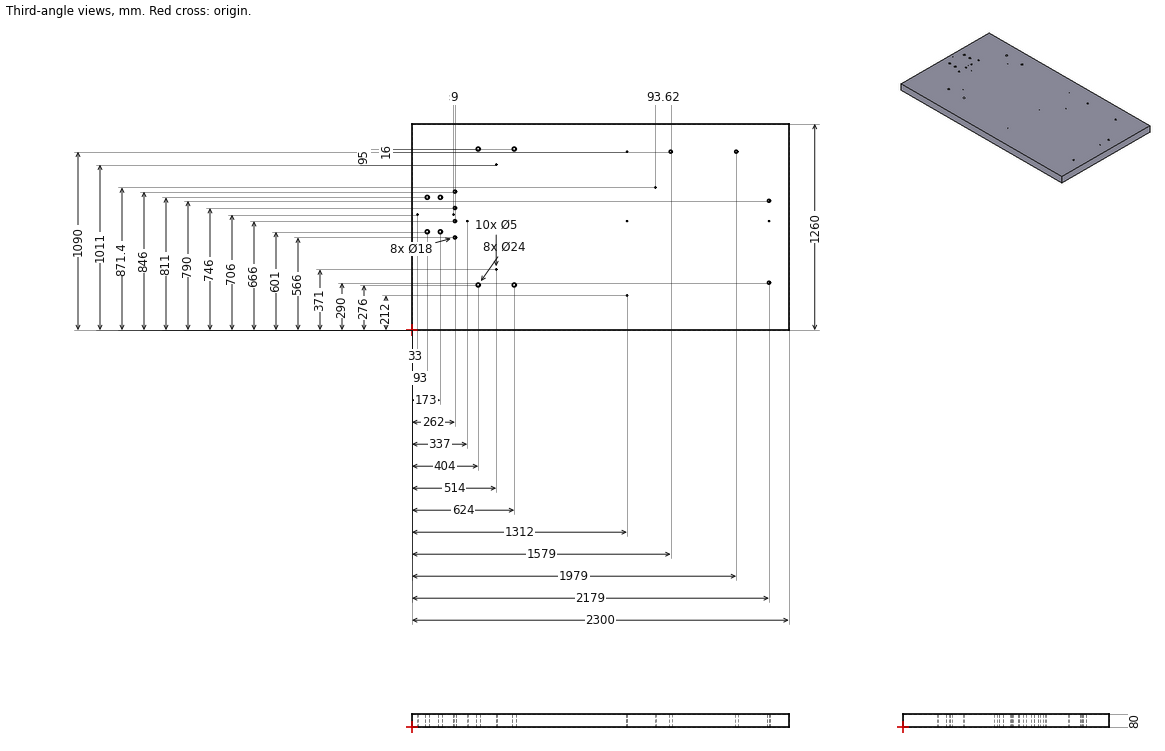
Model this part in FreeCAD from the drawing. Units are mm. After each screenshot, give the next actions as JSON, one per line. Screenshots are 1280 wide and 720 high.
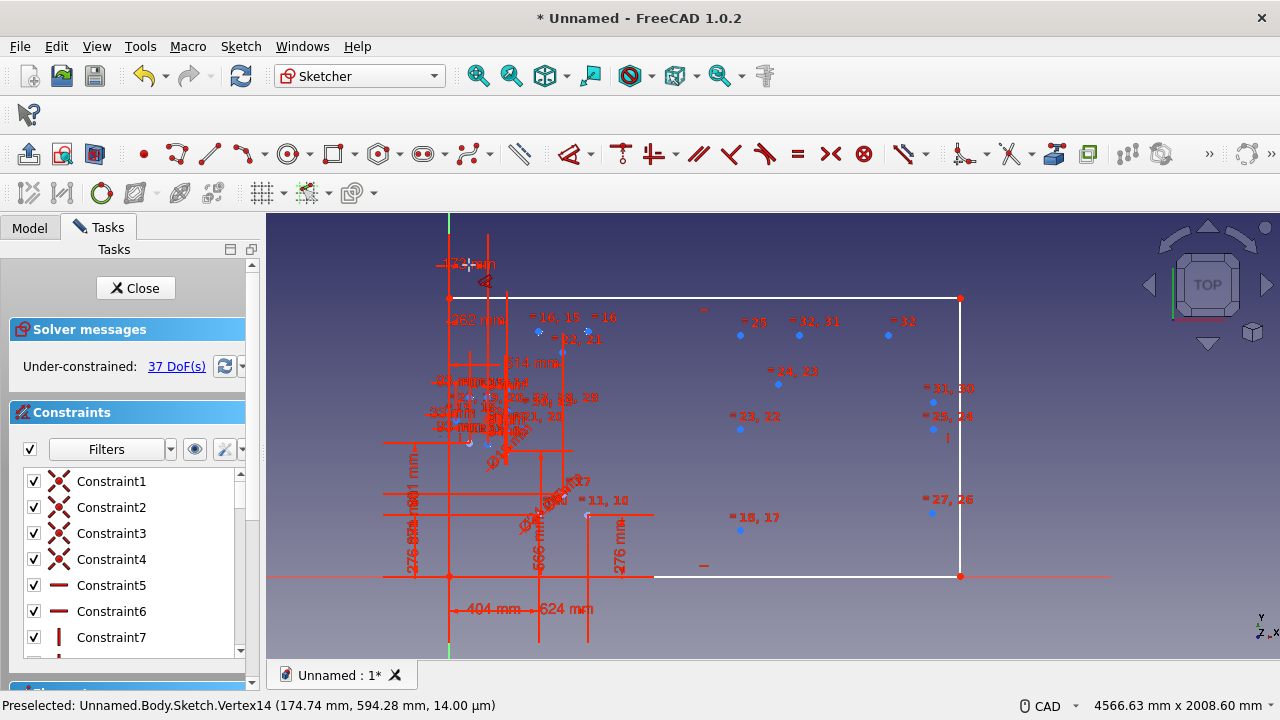
{"action": "left_click", "coordinate": [488, 445]}
{"action": "left_click", "coordinate": [343, 511]}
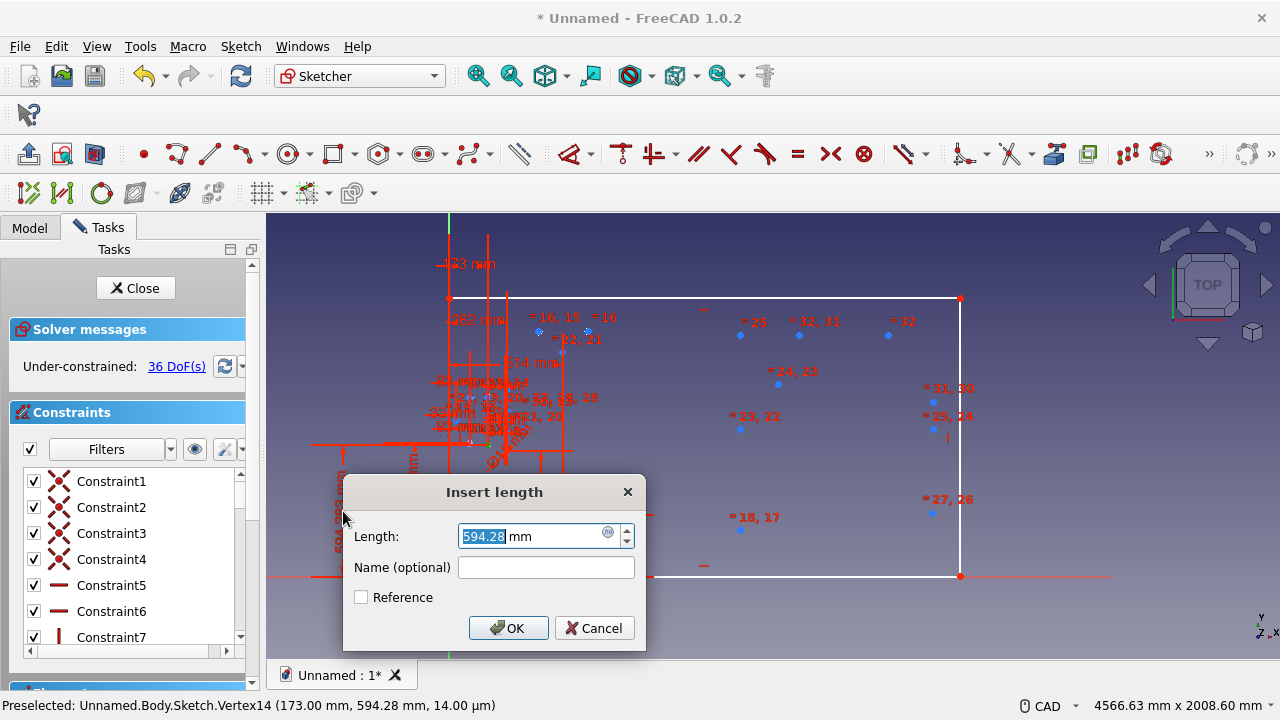
{"action": "type", "text": "601"}
{"action": "key", "text": "Return"}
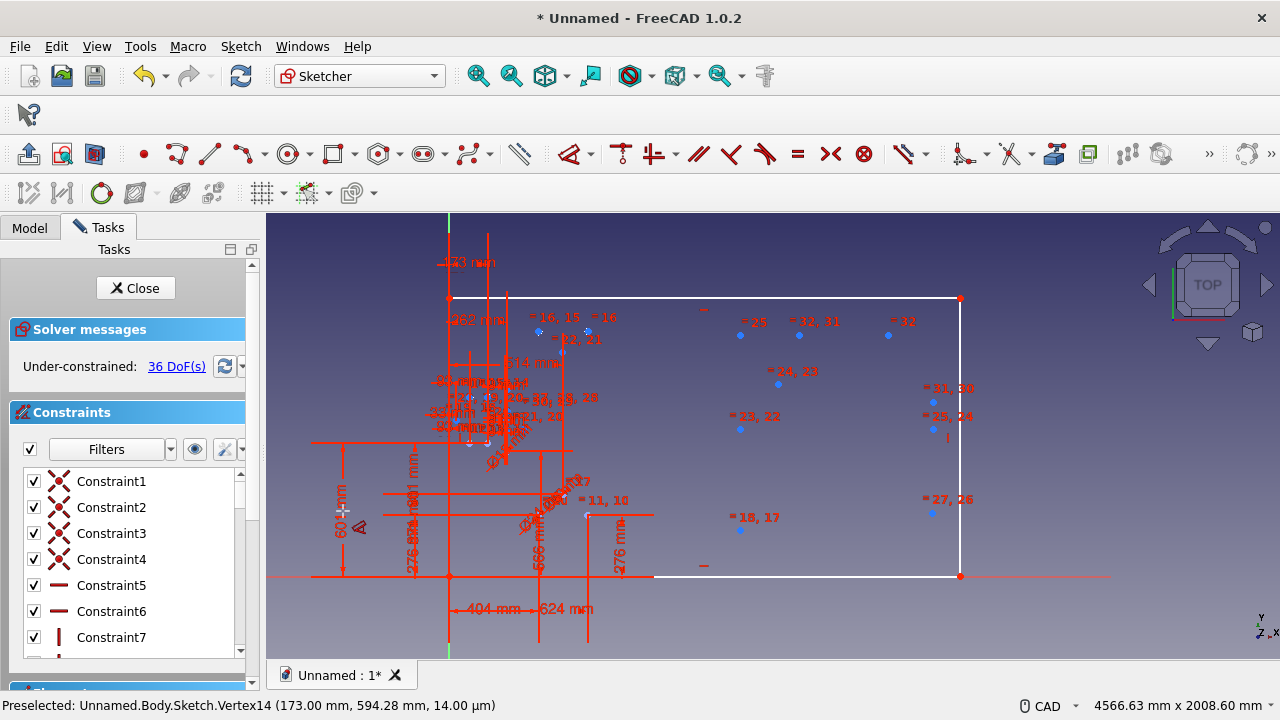
{"action": "left_click", "coordinate": [741, 530]}
{"action": "left_click", "coordinate": [775, 553]}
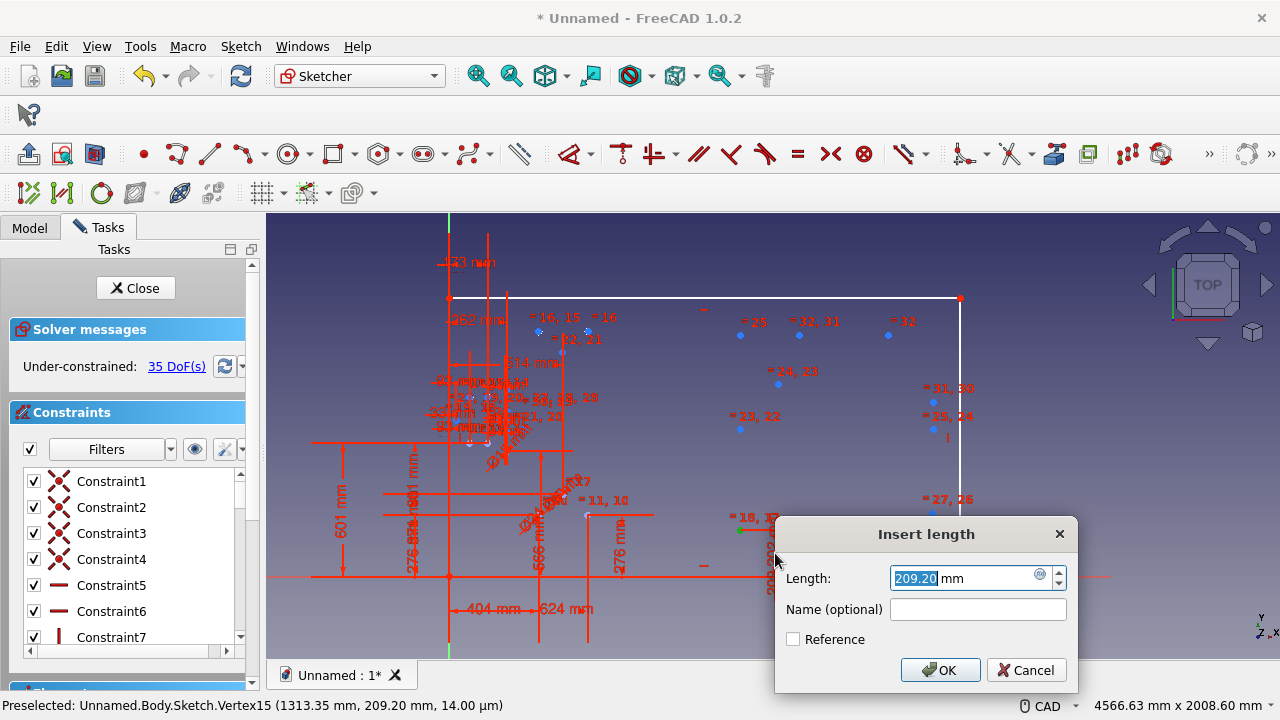
{"action": "type", "text": "212"}
{"action": "key", "text": "Return"}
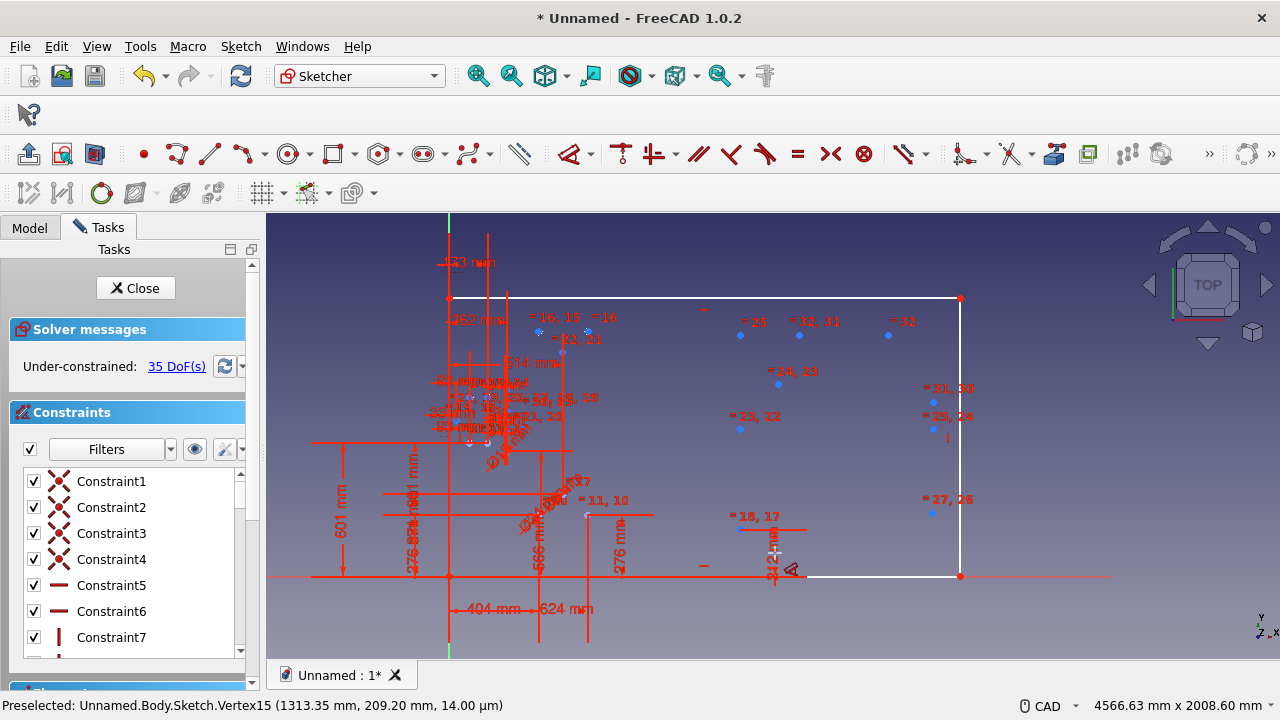
{"action": "left_click", "coordinate": [933, 513]}
{"action": "left_click", "coordinate": [991, 545]}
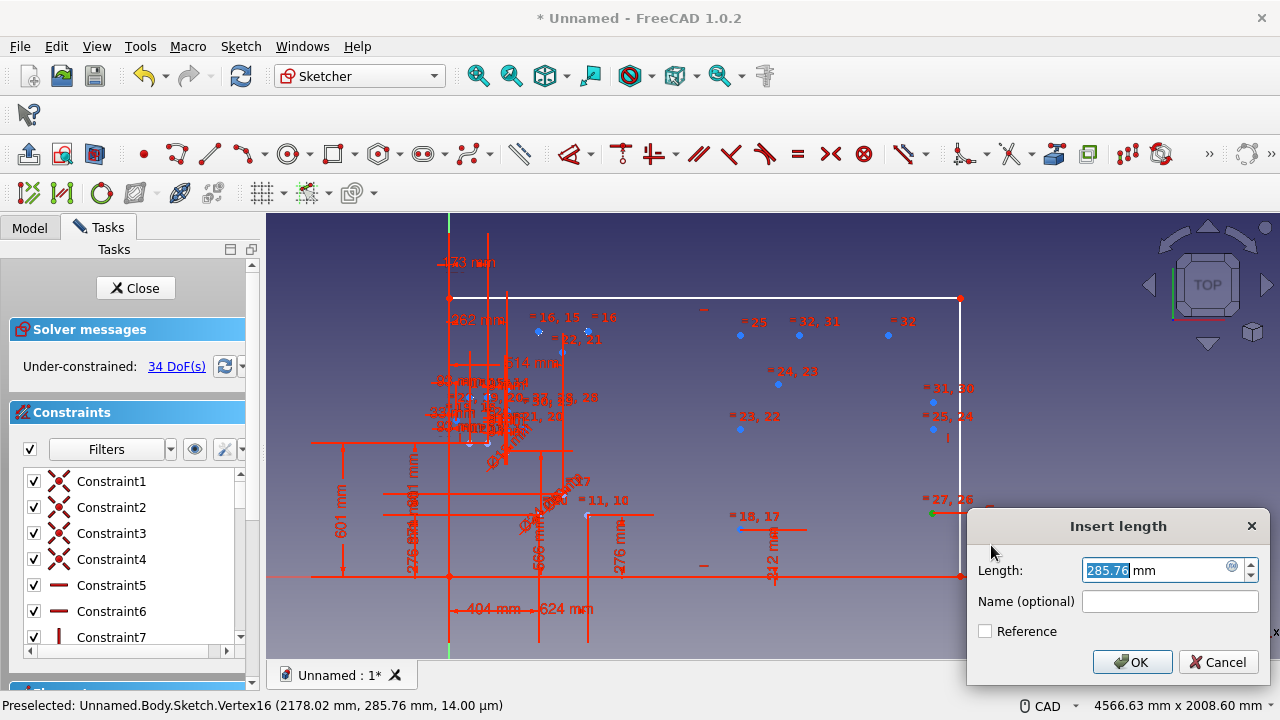
{"action": "type", "text": "290"}
{"action": "key", "text": "Return"}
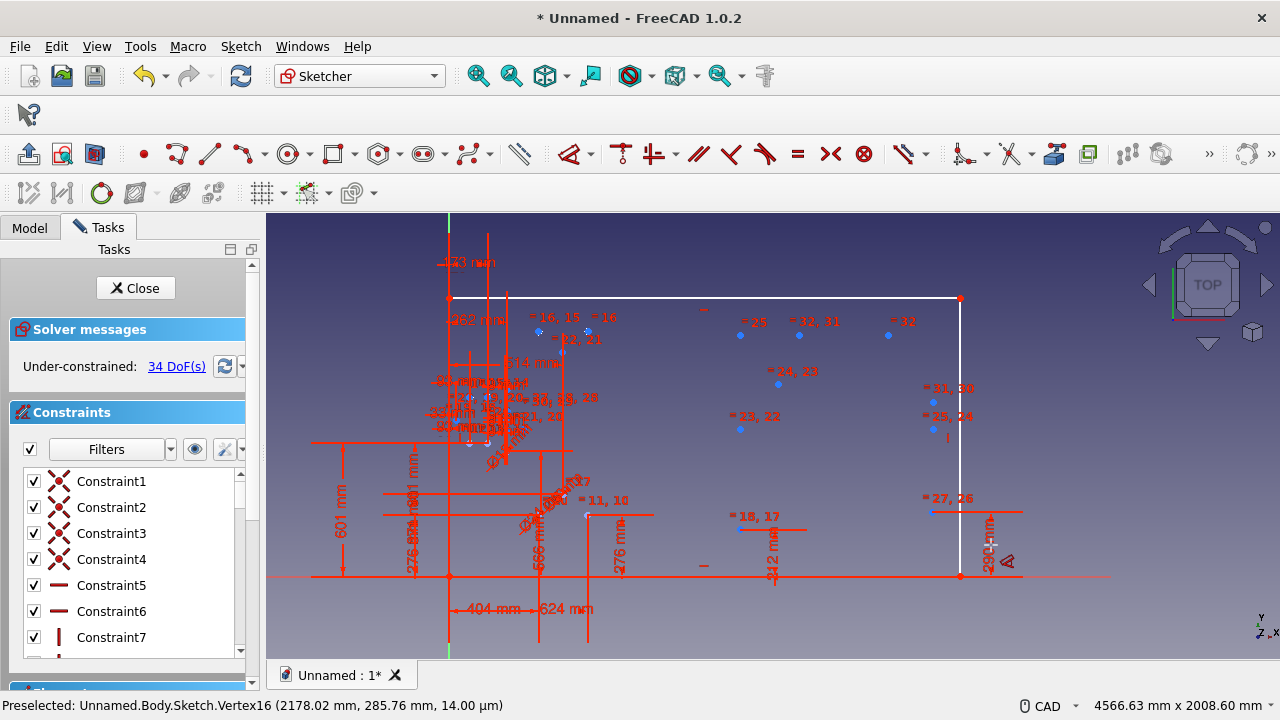
{"action": "left_click", "coordinate": [456, 420]}
{"action": "left_click", "coordinate": [367, 444]}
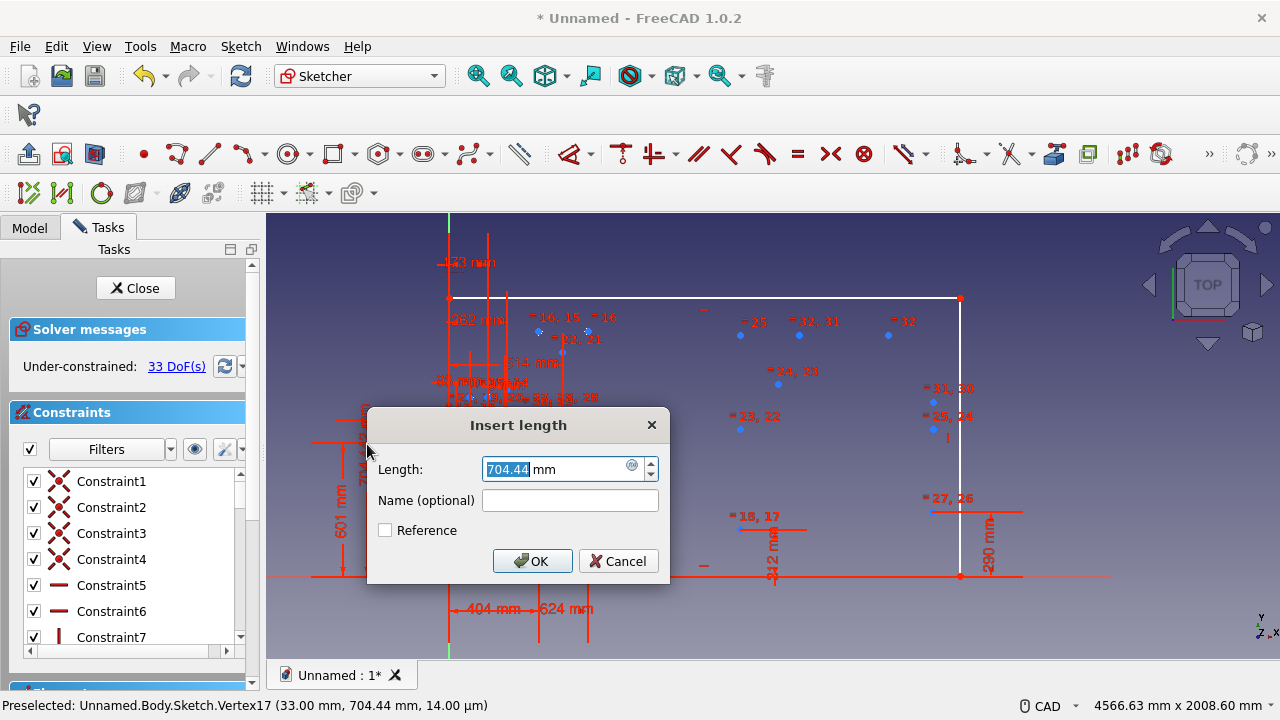
{"action": "type", "text": "706"}
{"action": "key", "text": "Return"}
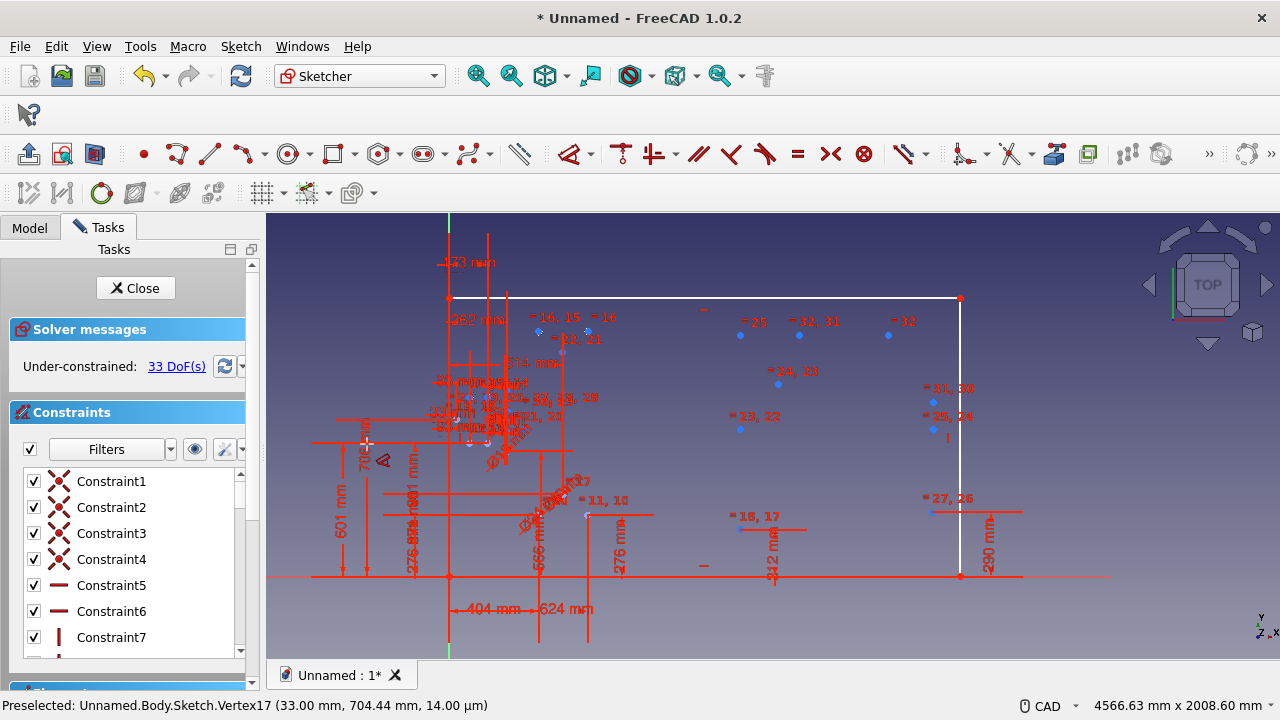
{"action": "left_click", "coordinate": [507, 430]}
{"action": "left_click", "coordinate": [541, 470]}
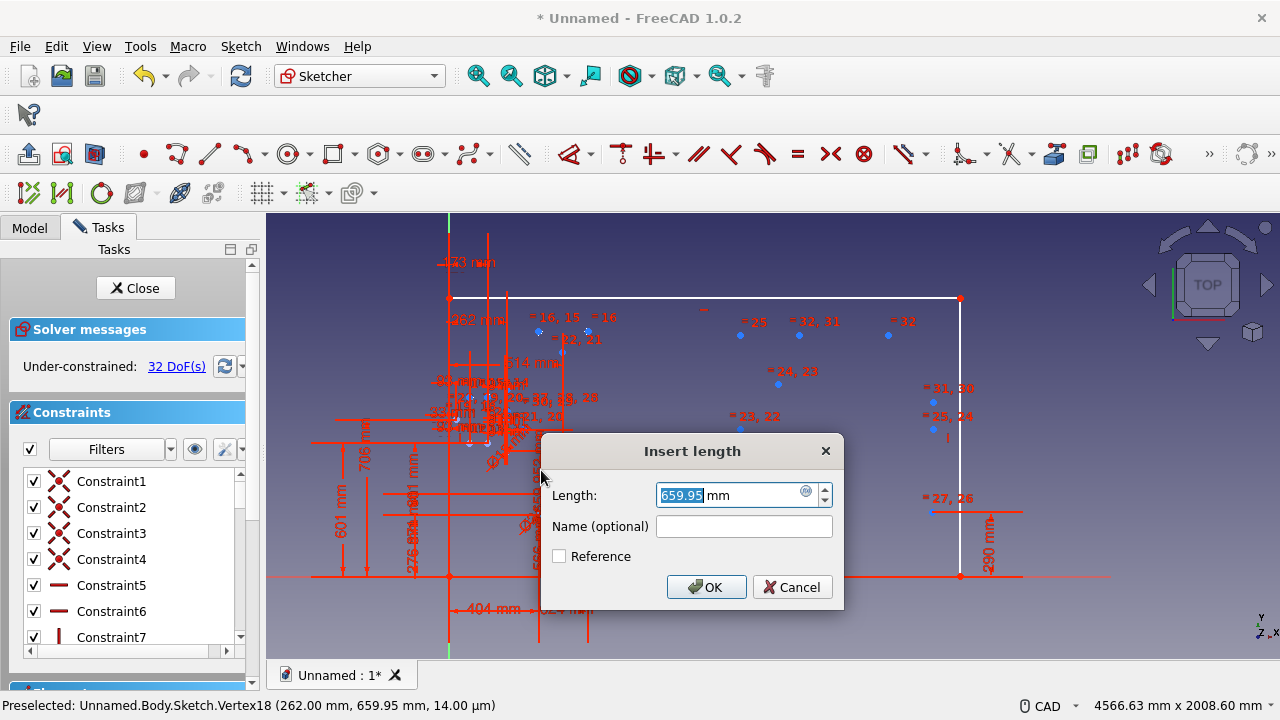
{"action": "type", "text": "666"}
{"action": "key", "text": "Return"}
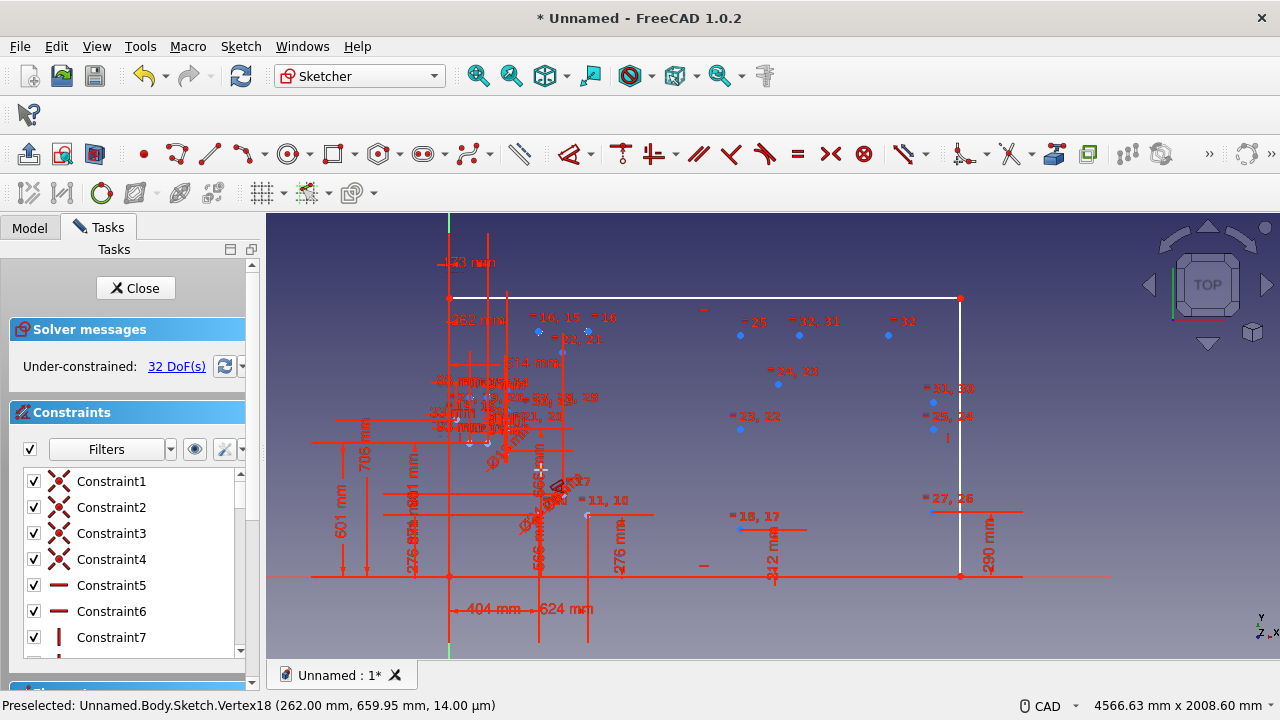
{"action": "scroll", "coordinate": [505, 420], "scroll_direction": "up", "scroll_amount": 2}